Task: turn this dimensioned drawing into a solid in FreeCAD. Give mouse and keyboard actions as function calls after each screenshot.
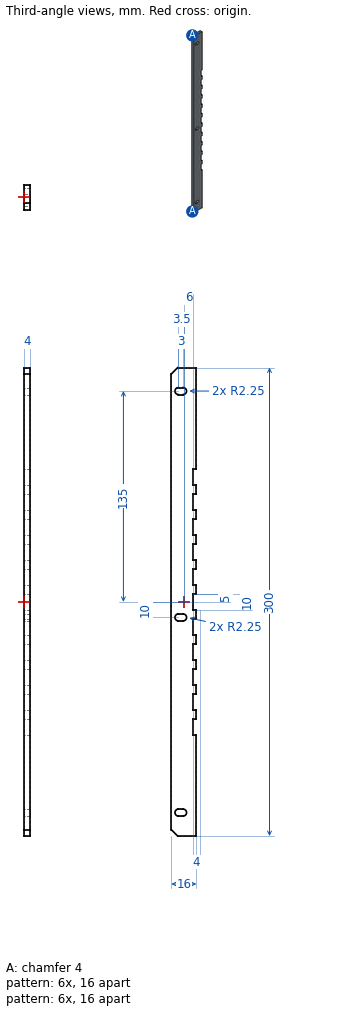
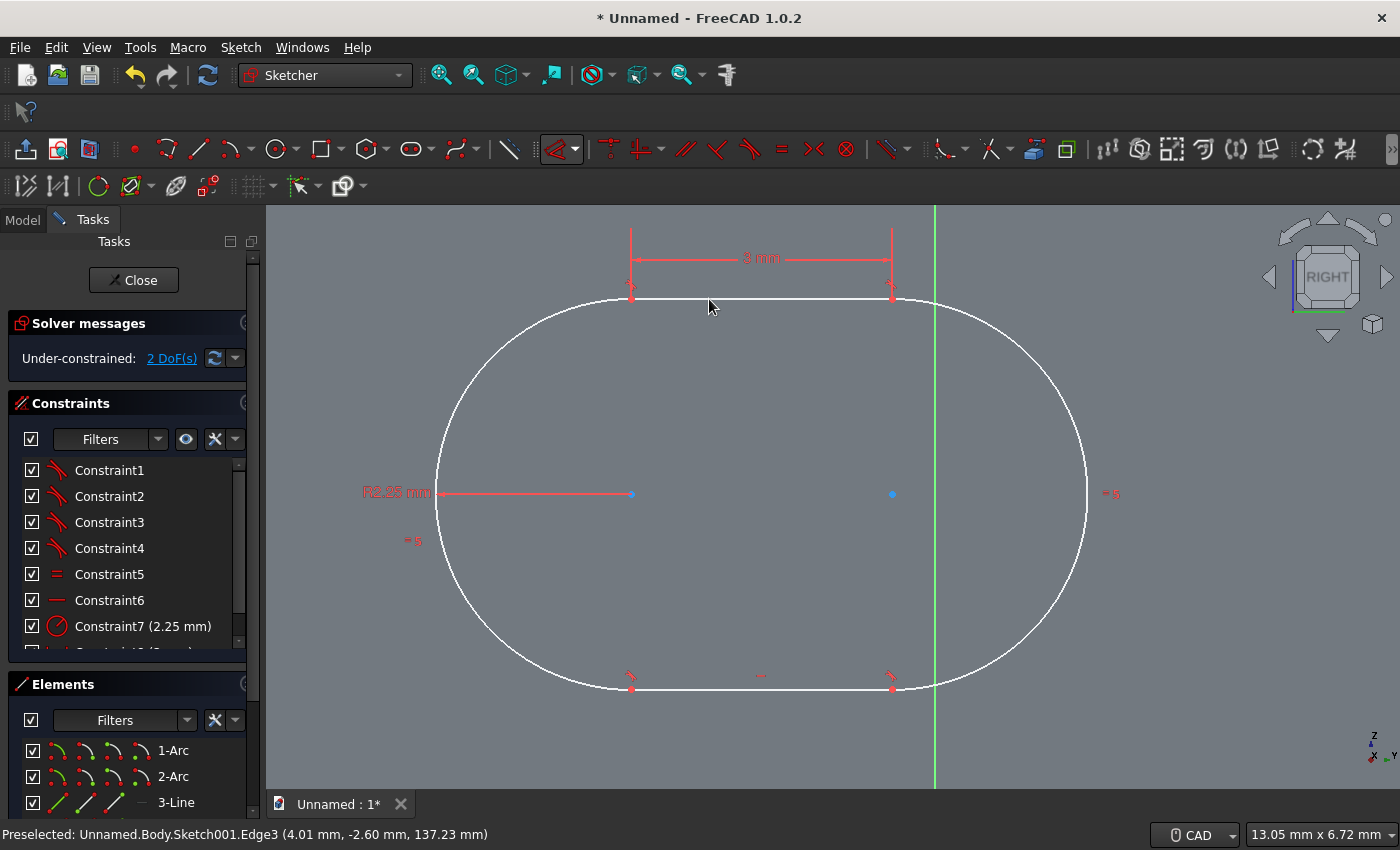
click(631, 299)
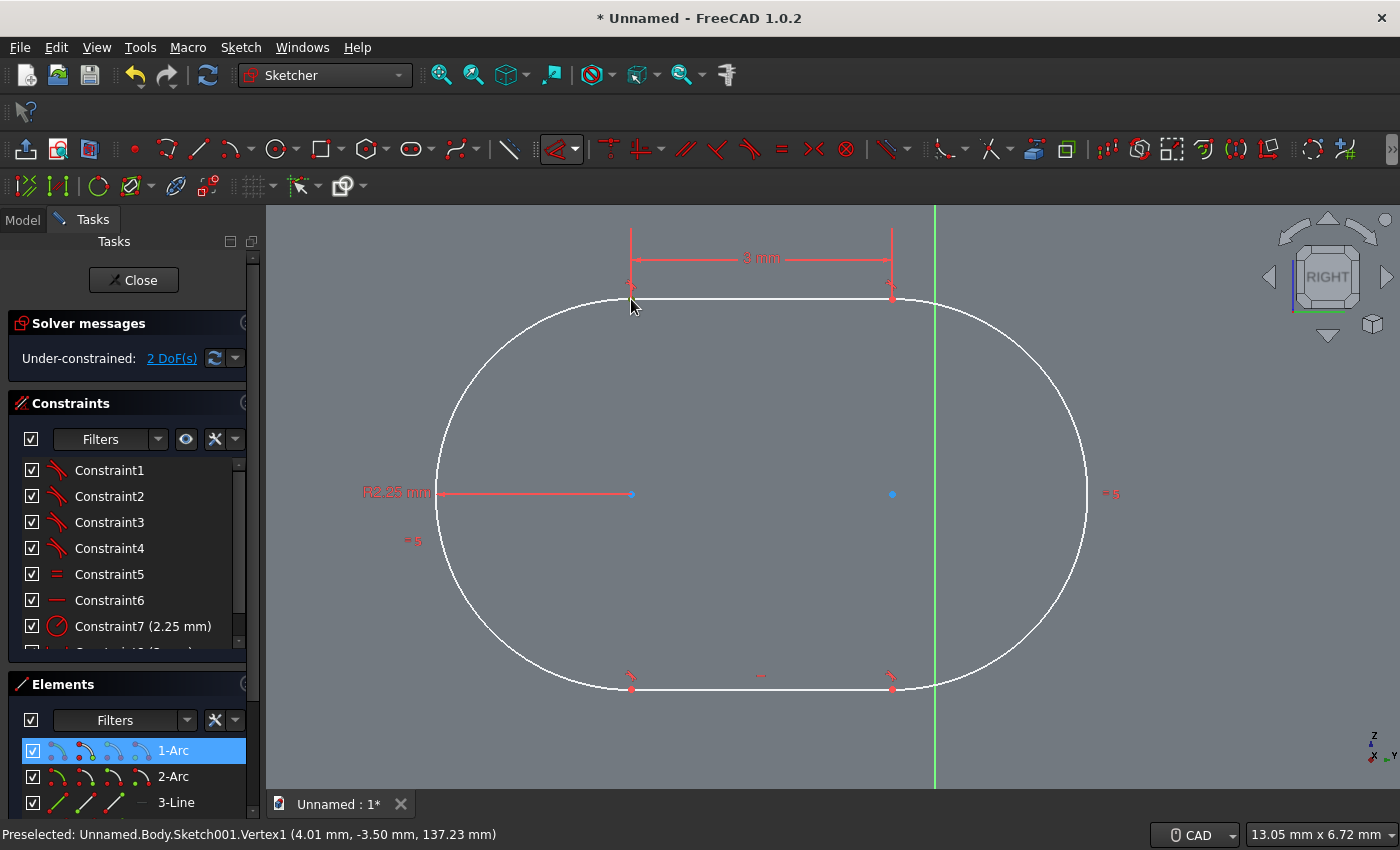
key(l)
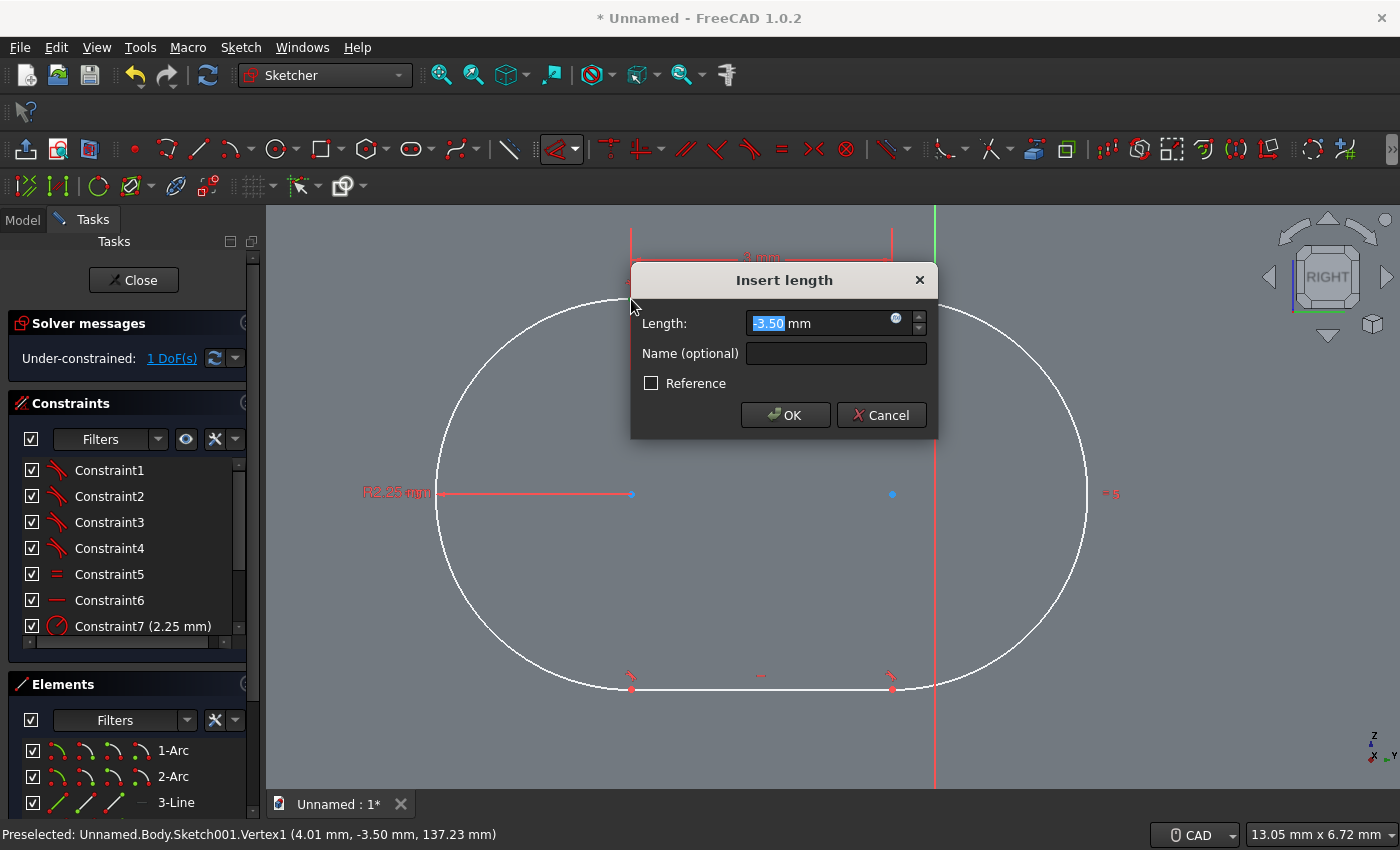
text(-3.5)
key(Return)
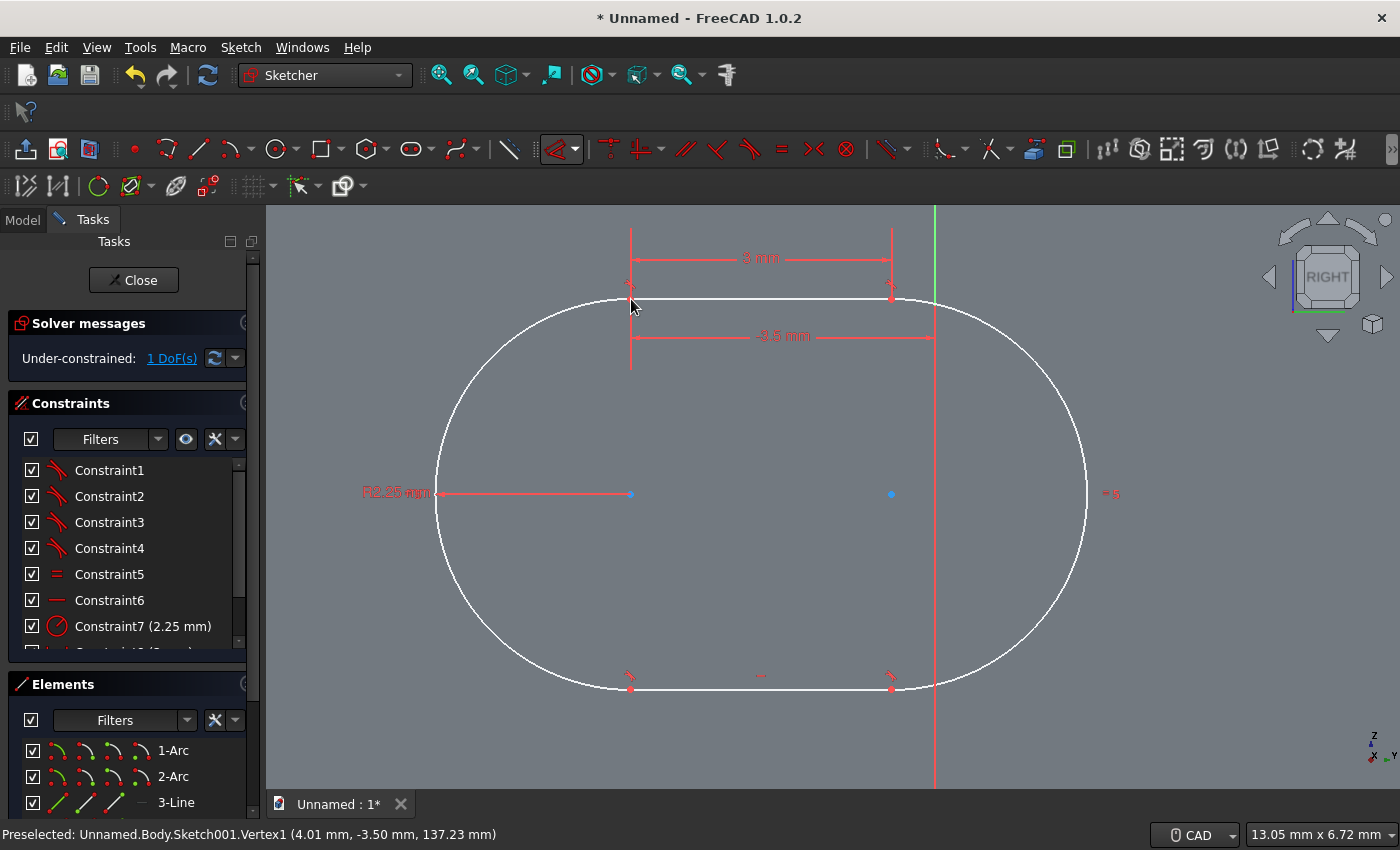
click(631, 494)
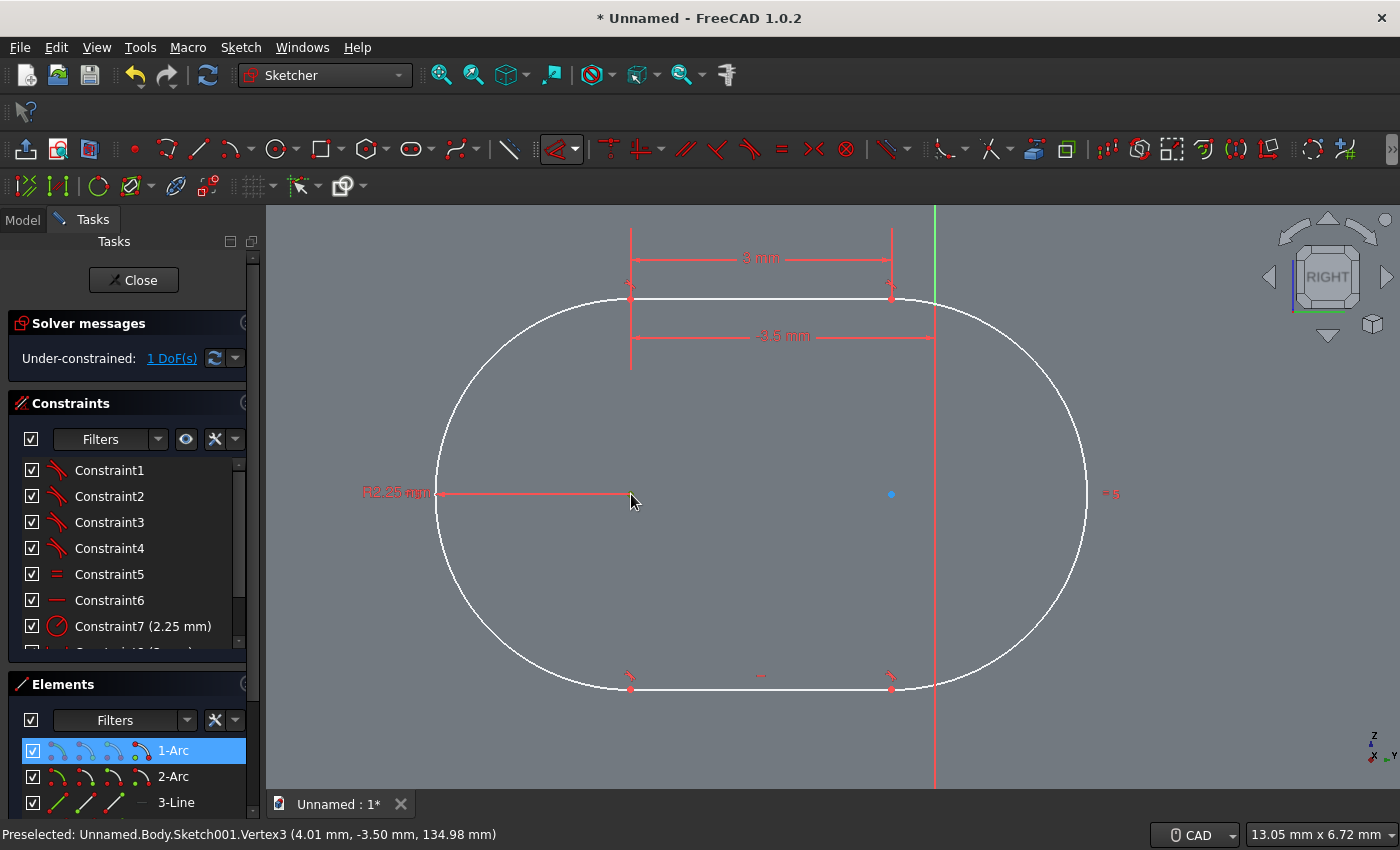
key(i)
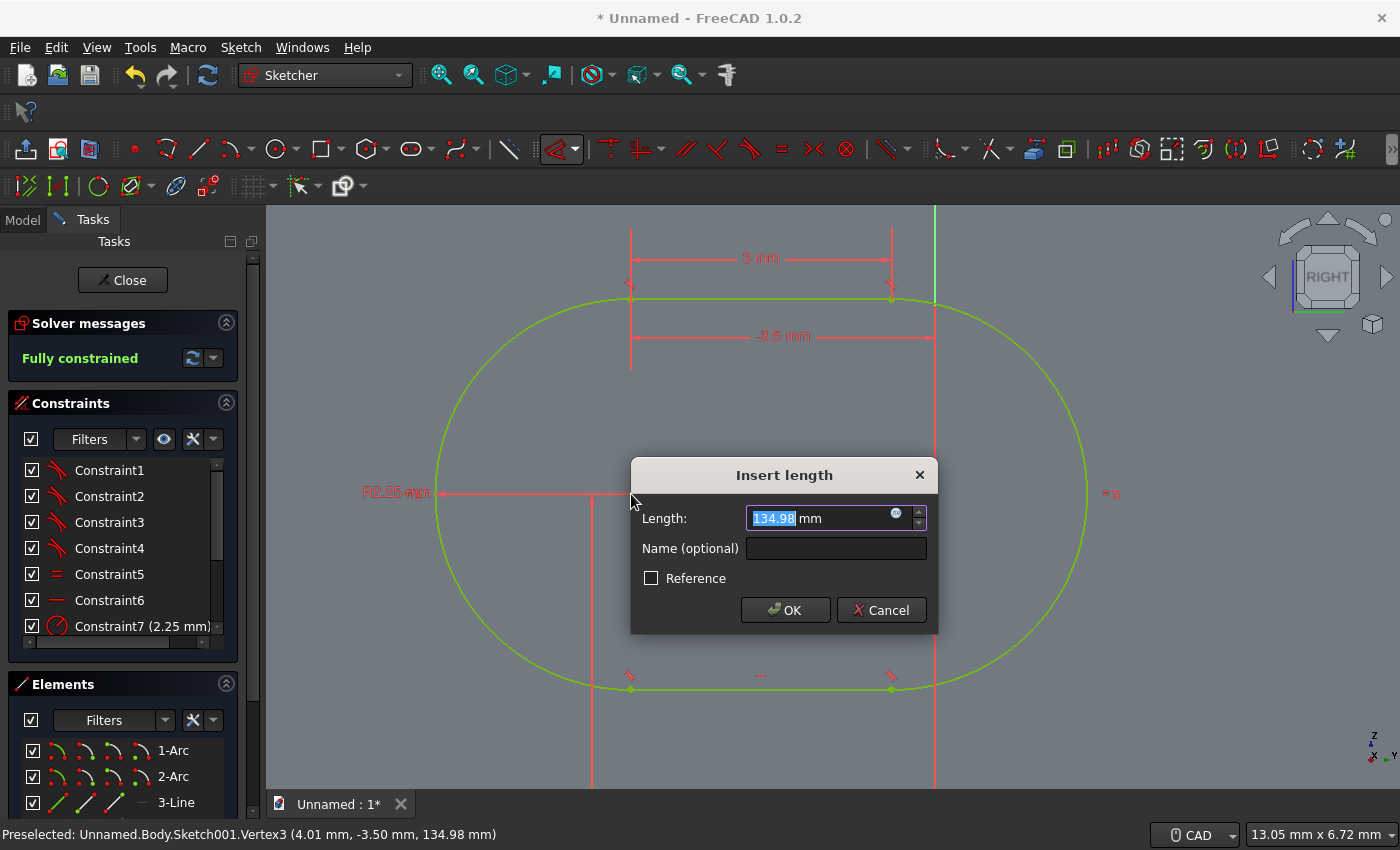
text(135)
key(Return)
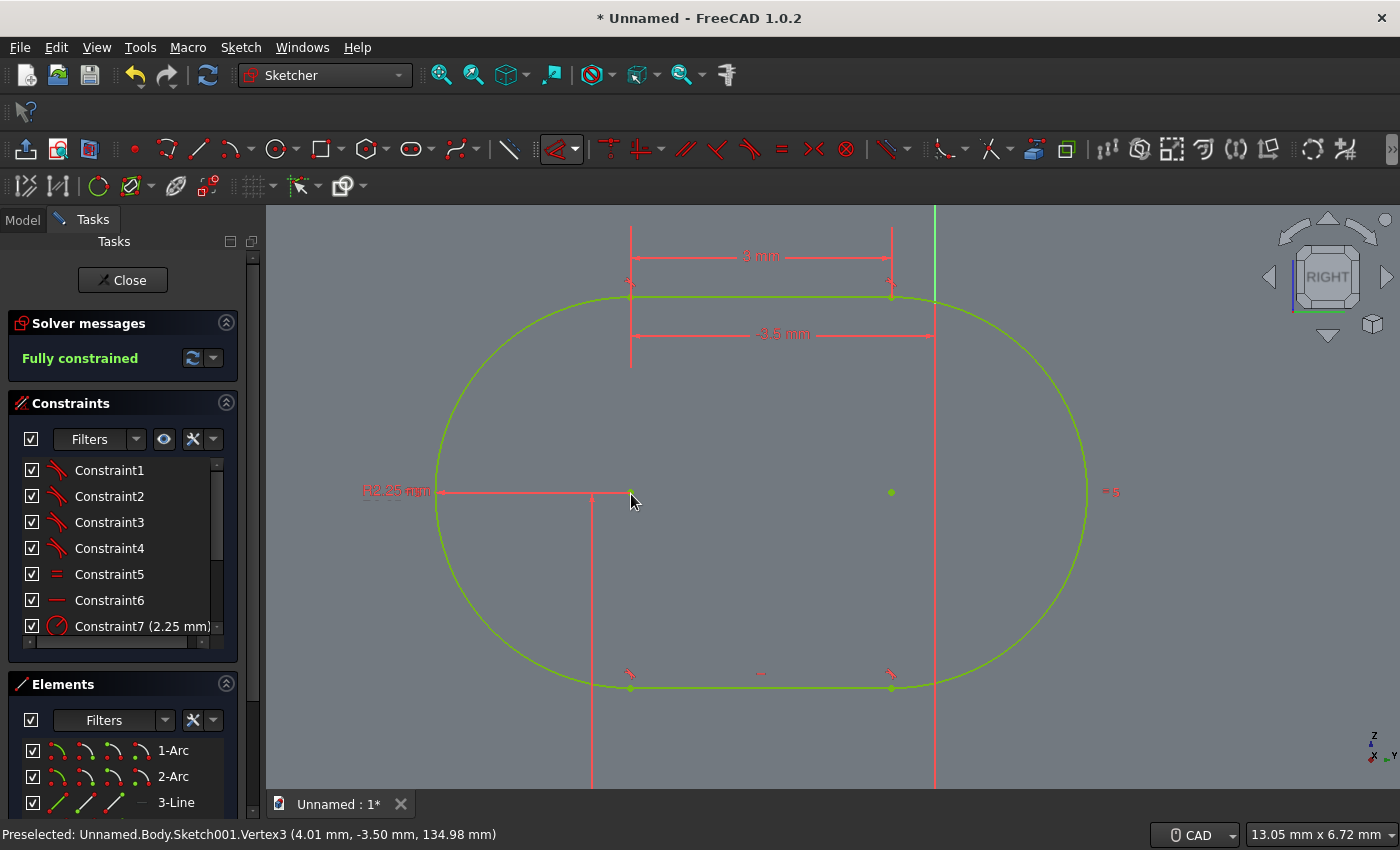
click(123, 280)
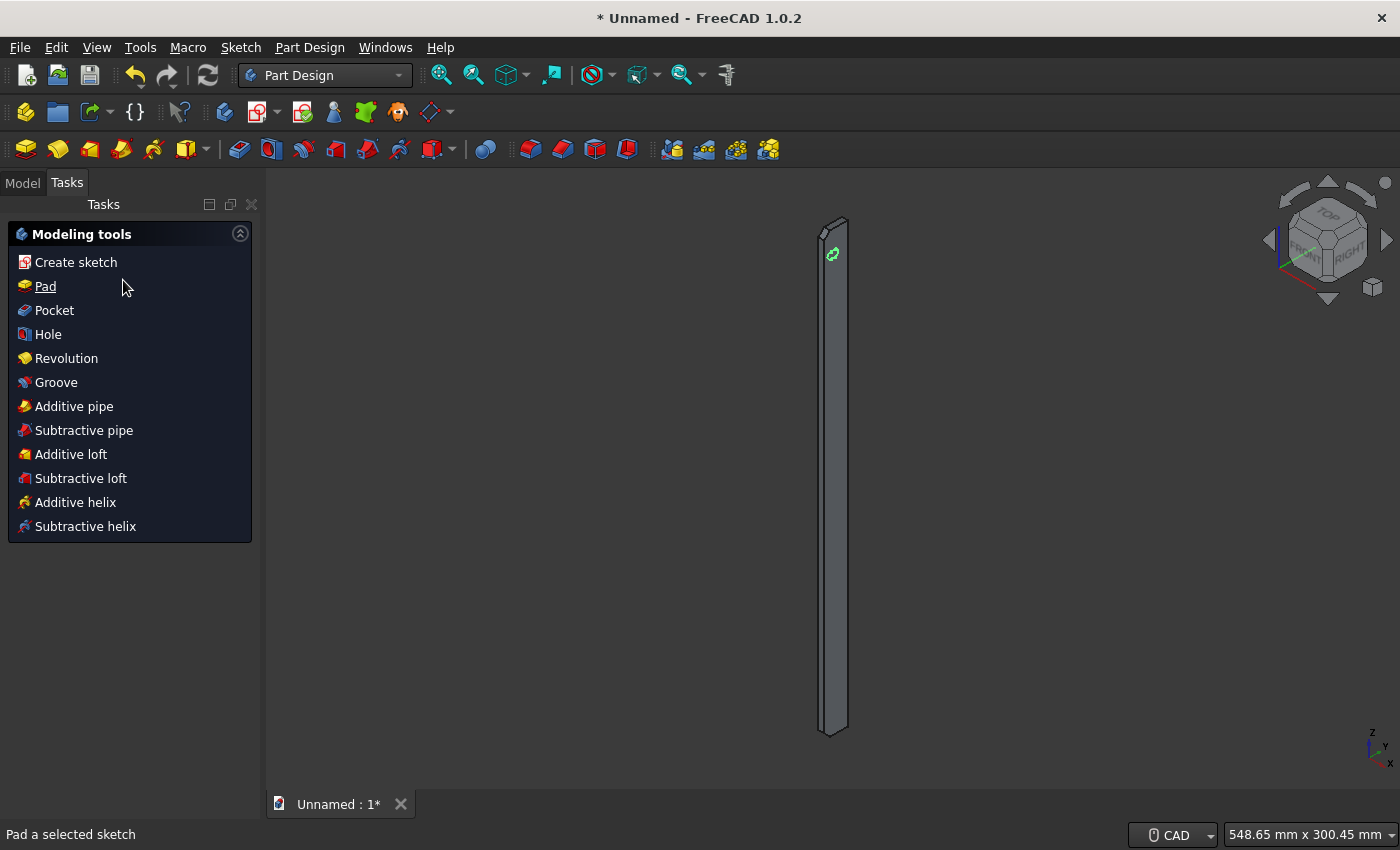
click(240, 150)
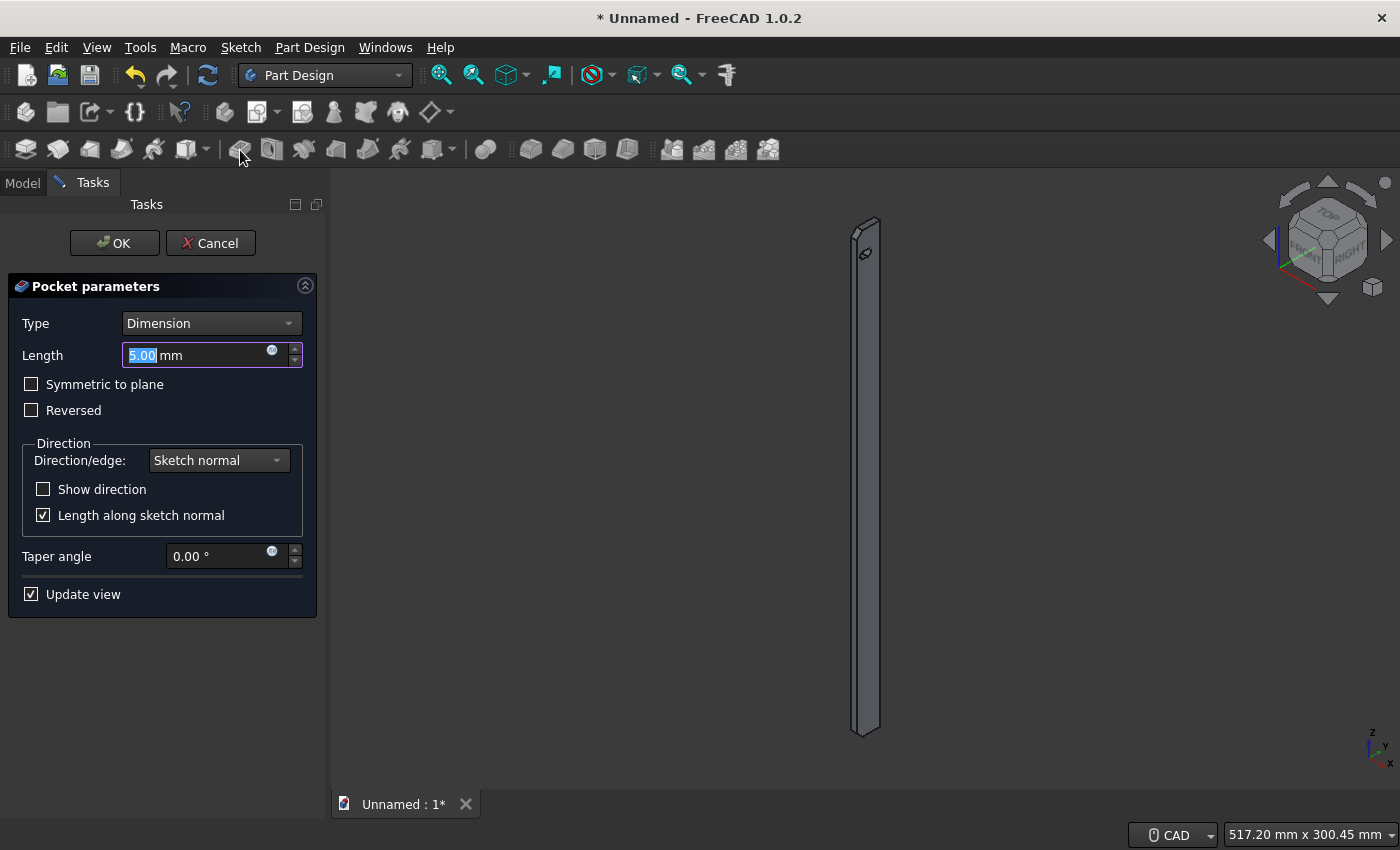
click(212, 324)